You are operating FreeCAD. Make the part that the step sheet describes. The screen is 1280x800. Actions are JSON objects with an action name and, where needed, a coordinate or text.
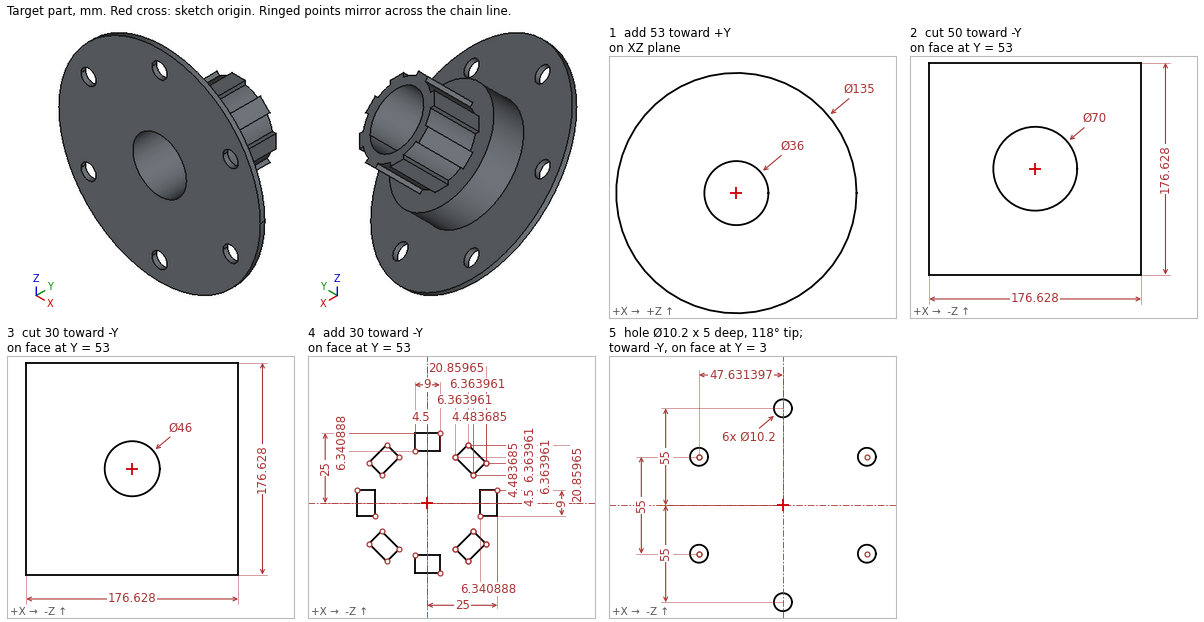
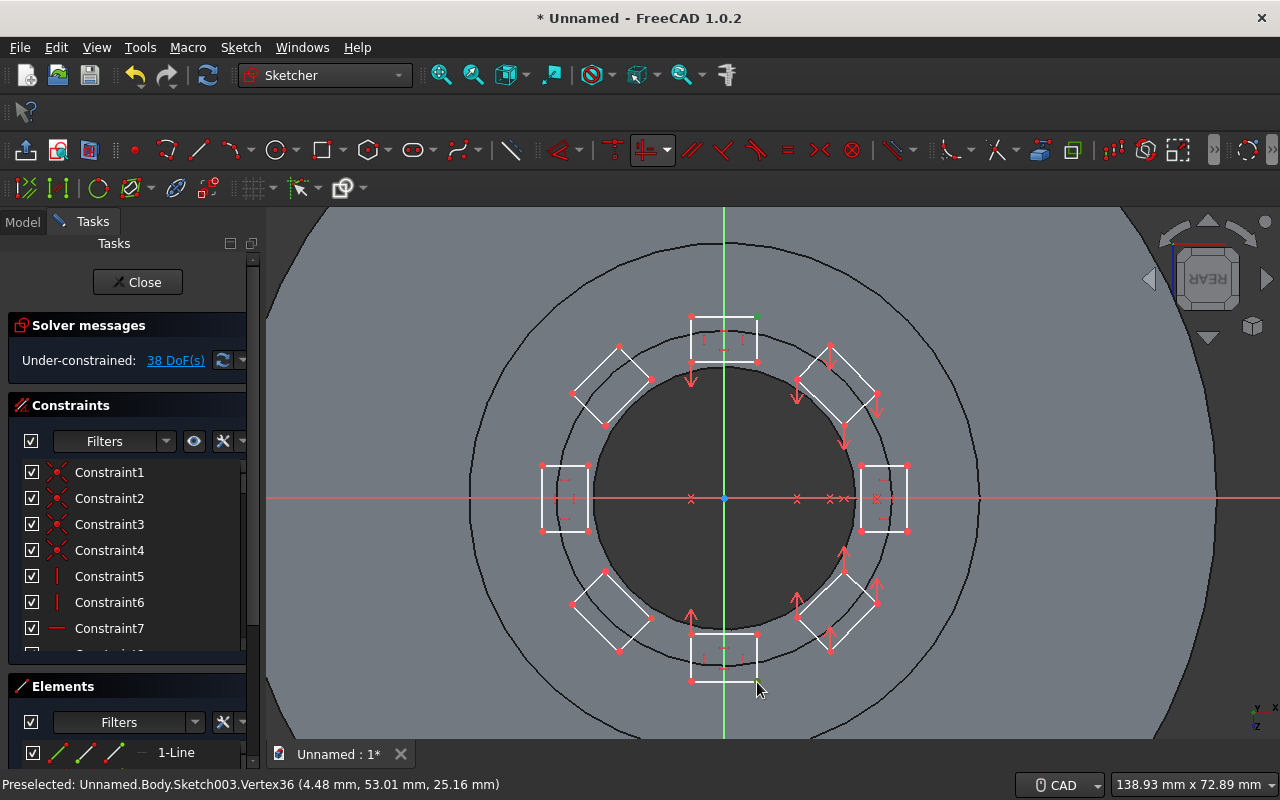
{"action": "left_click", "coordinate": [353, 498]}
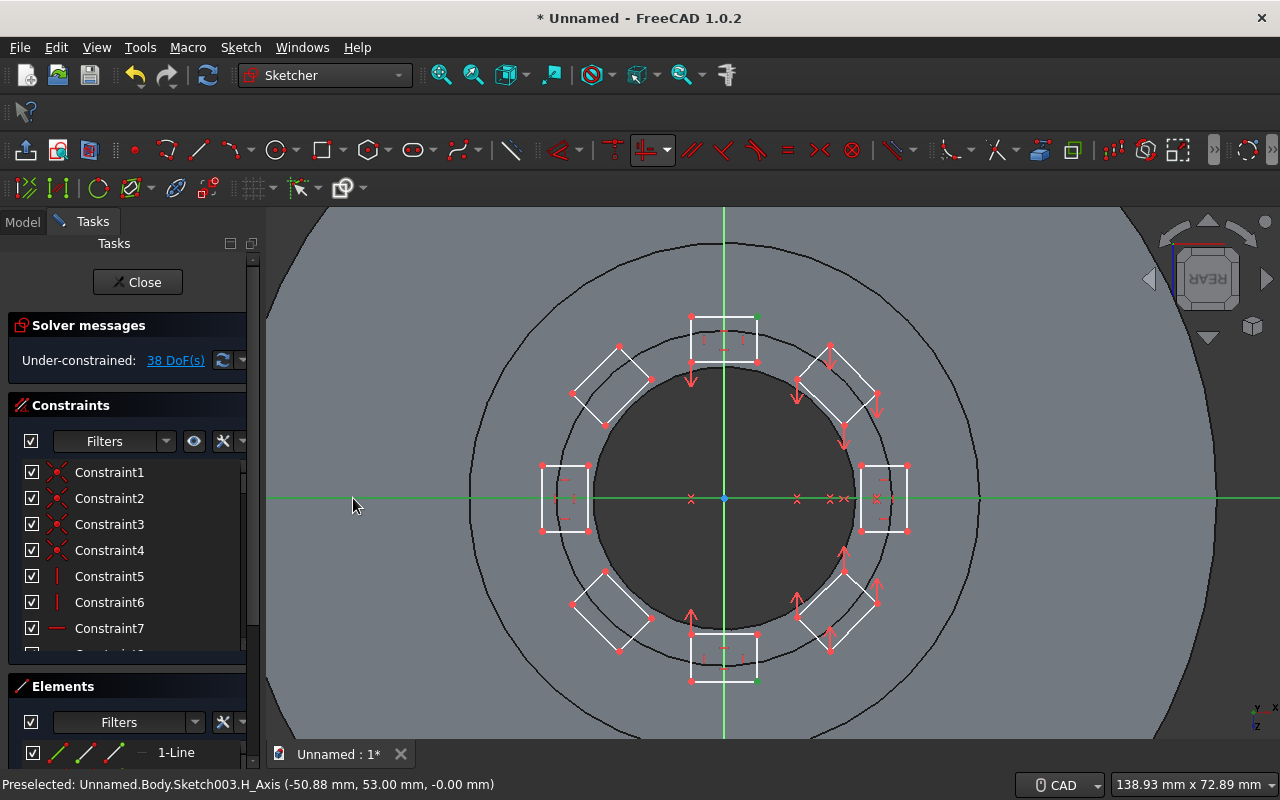
{"action": "left_click", "coordinate": [820, 150]}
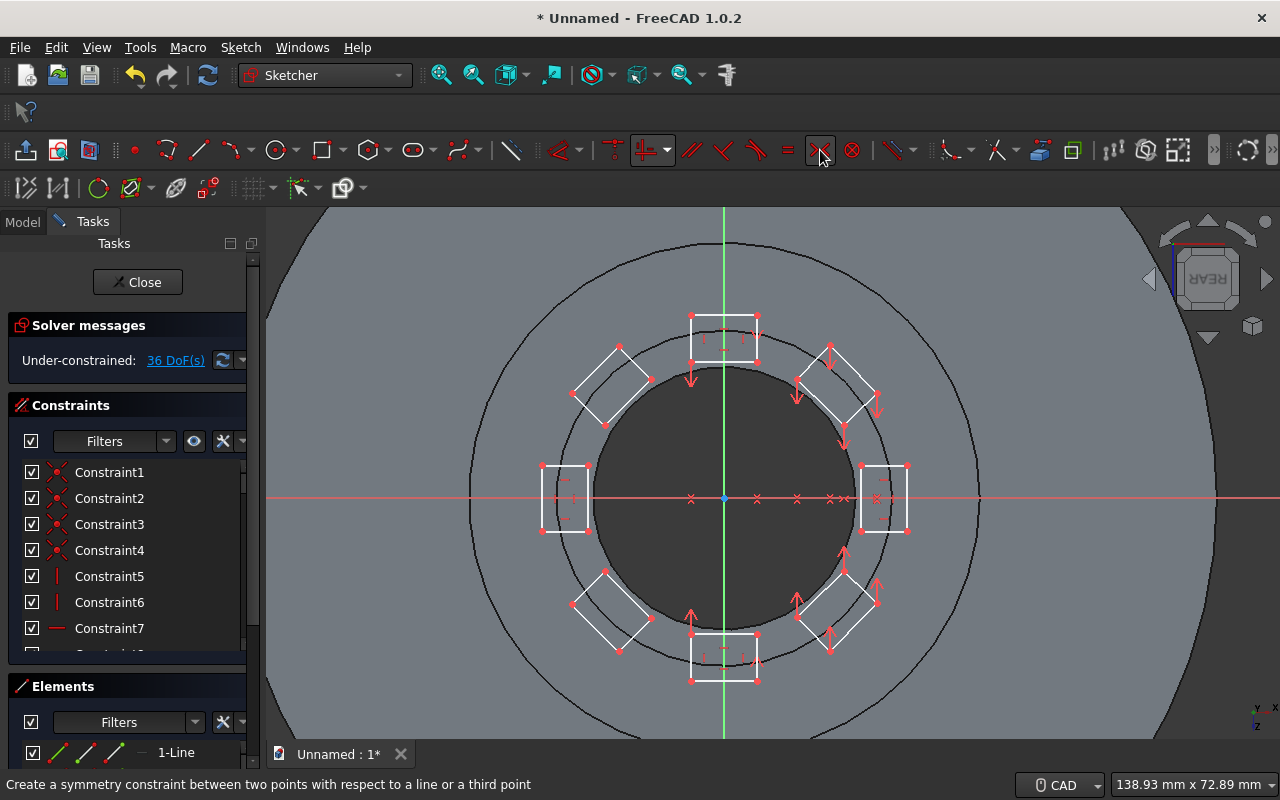
{"action": "left_click", "coordinate": [797, 617]}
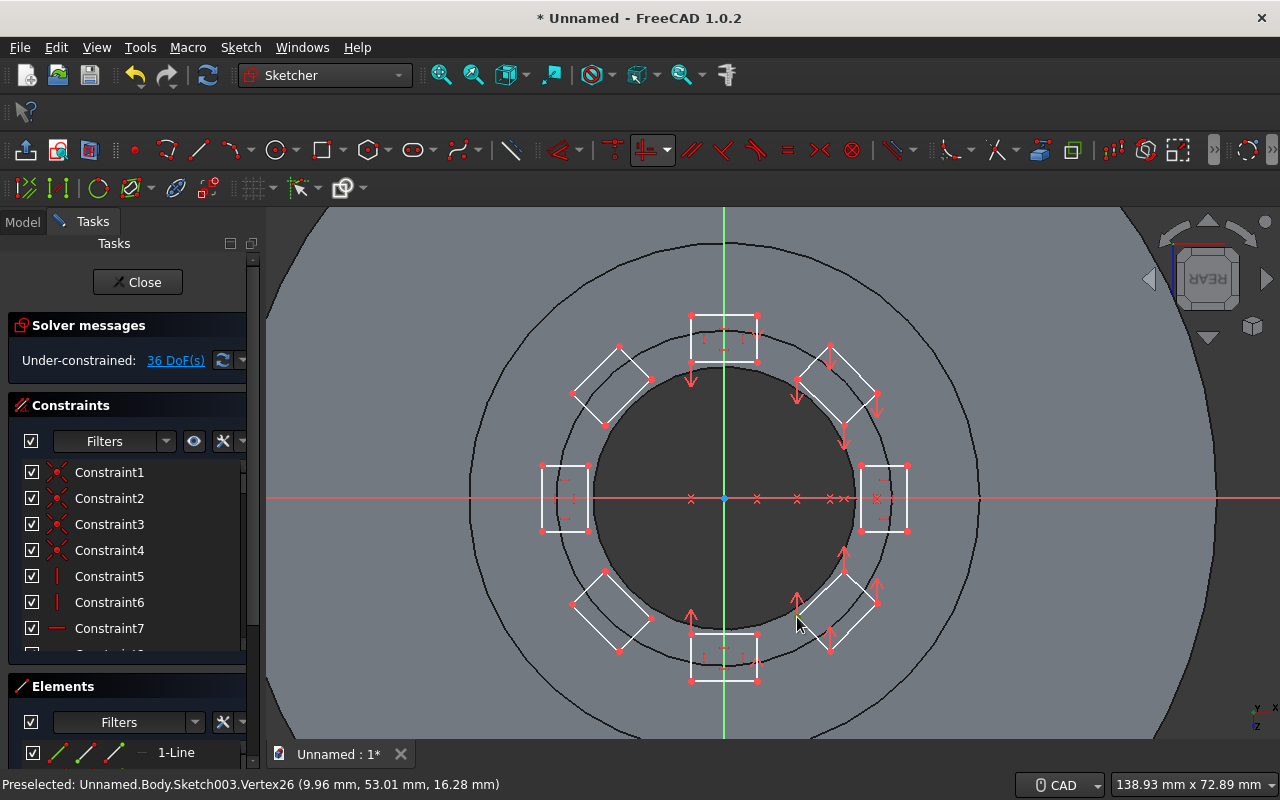
{"action": "left_click", "coordinate": [651, 619]}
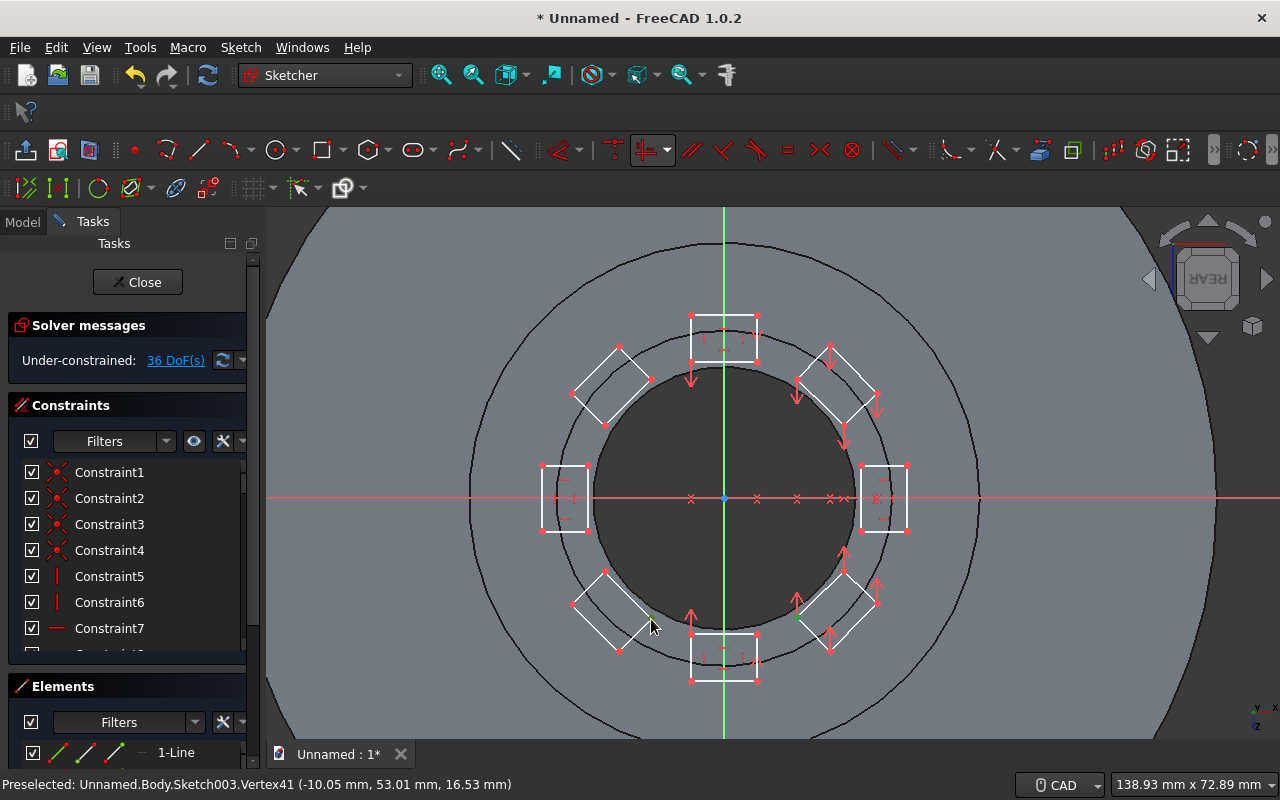
{"action": "left_click", "coordinate": [724, 575]}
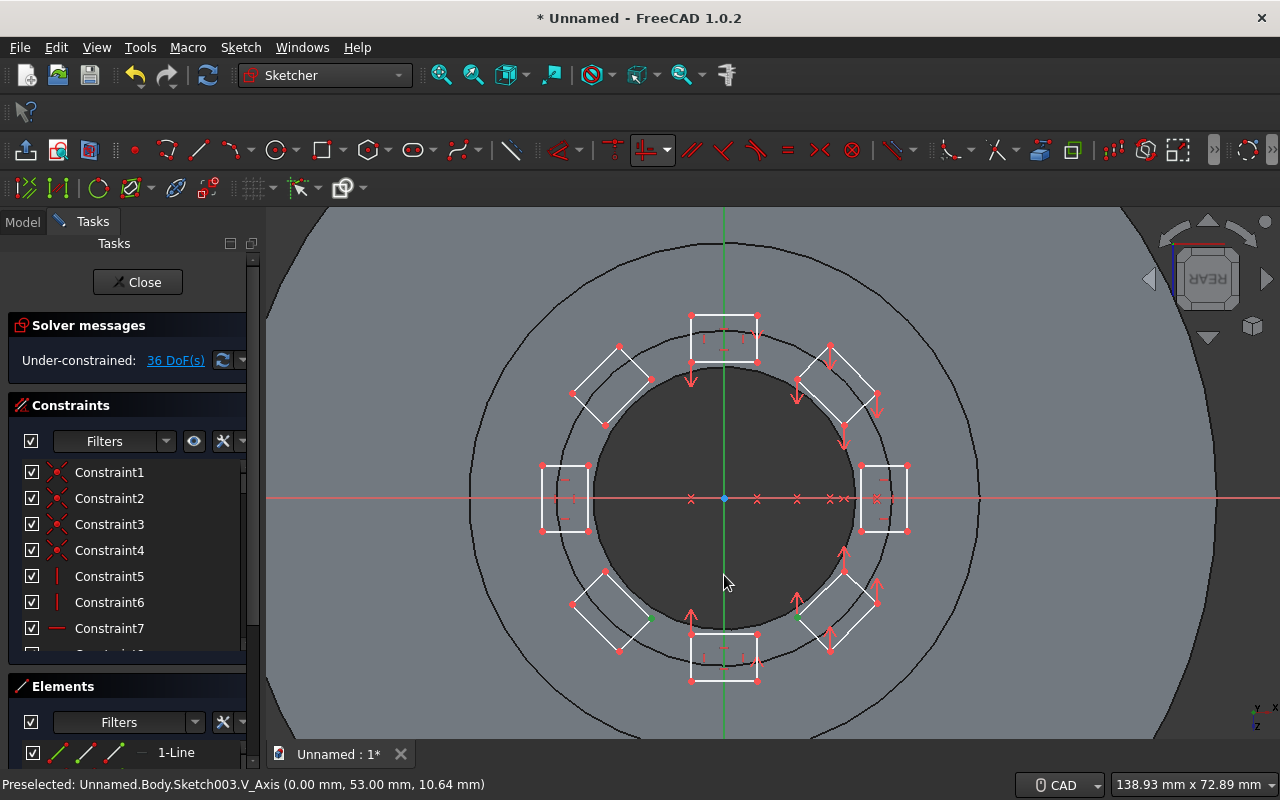
{"action": "left_click", "coordinate": [820, 150]}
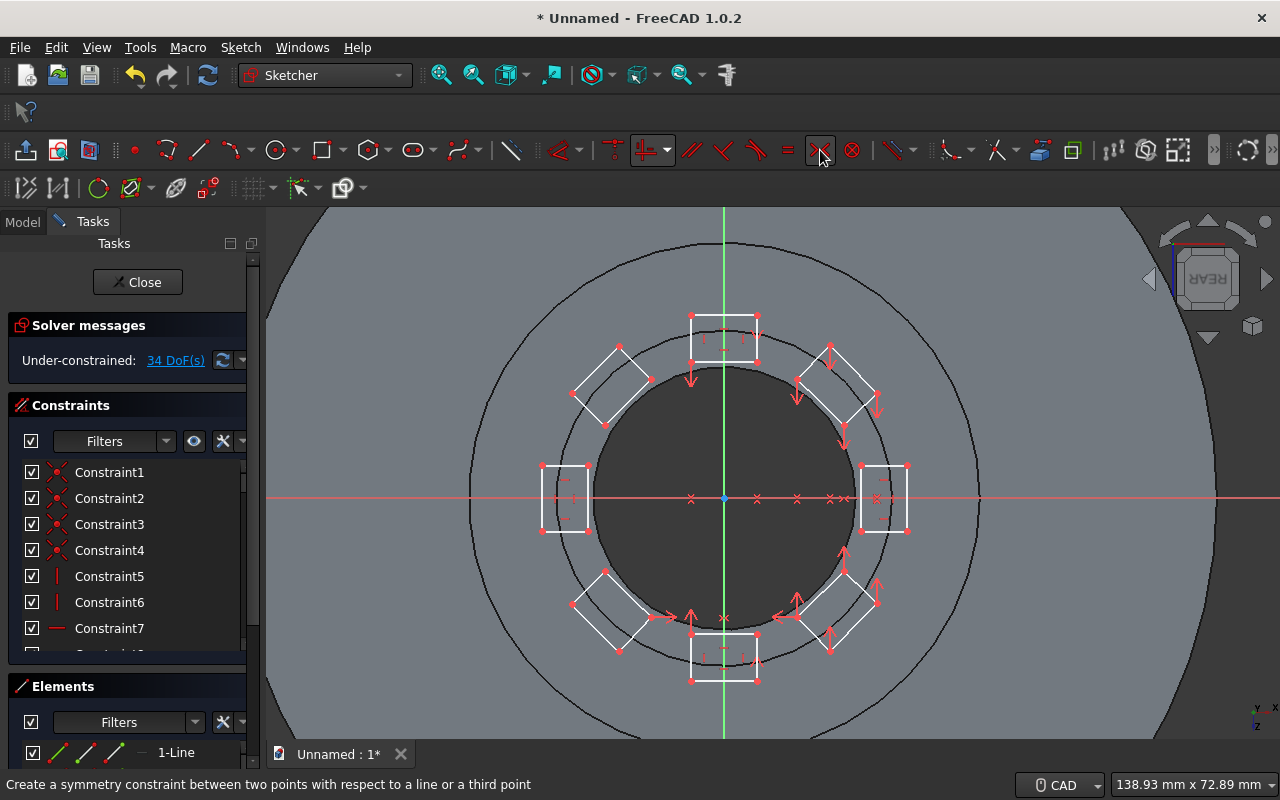
{"action": "left_click", "coordinate": [844, 571]}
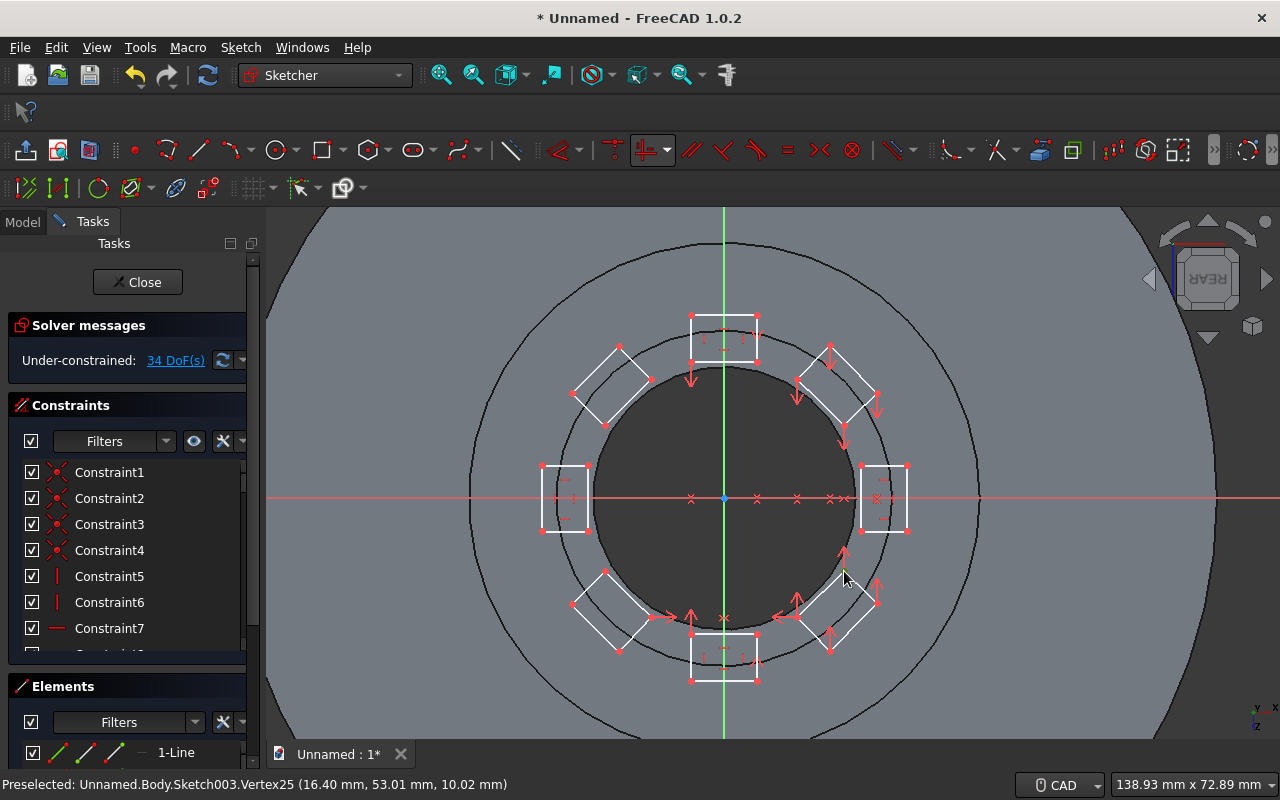
{"action": "left_click", "coordinate": [605, 572]}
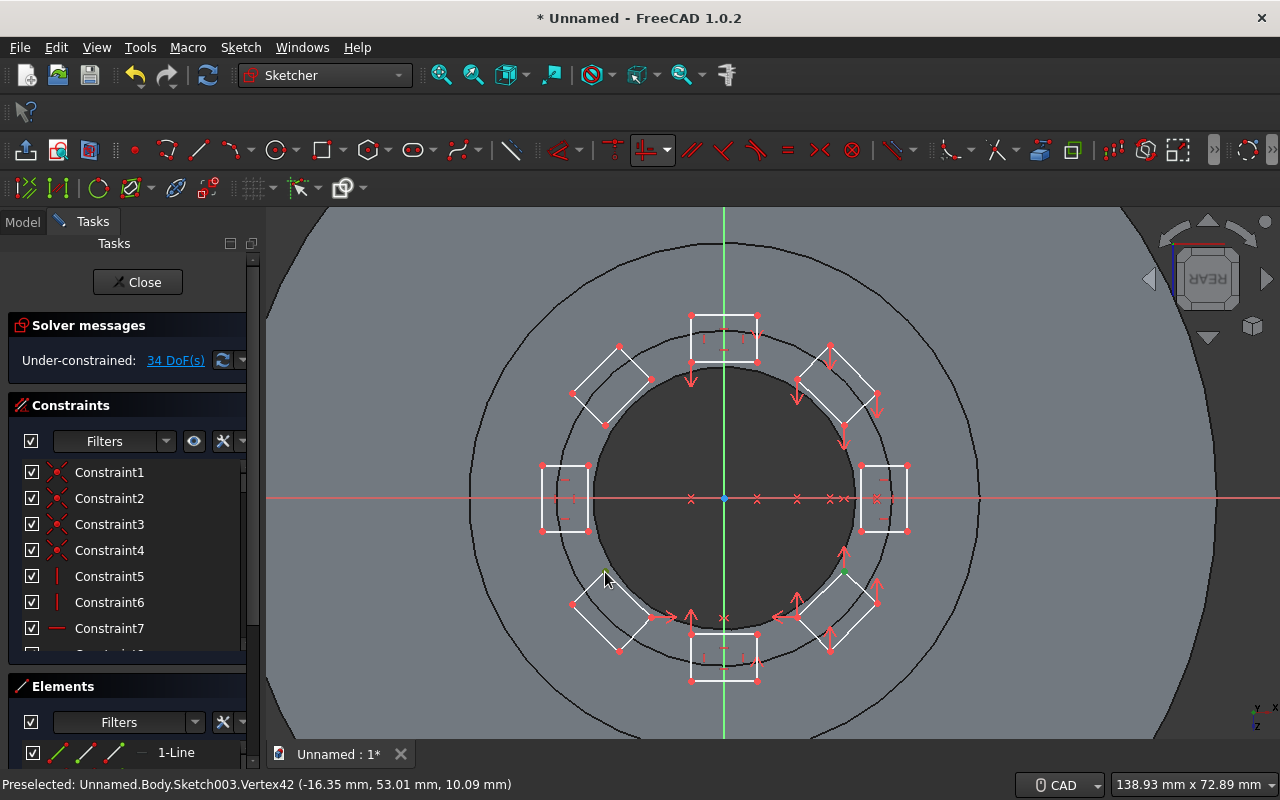
{"action": "left_click", "coordinate": [724, 575]}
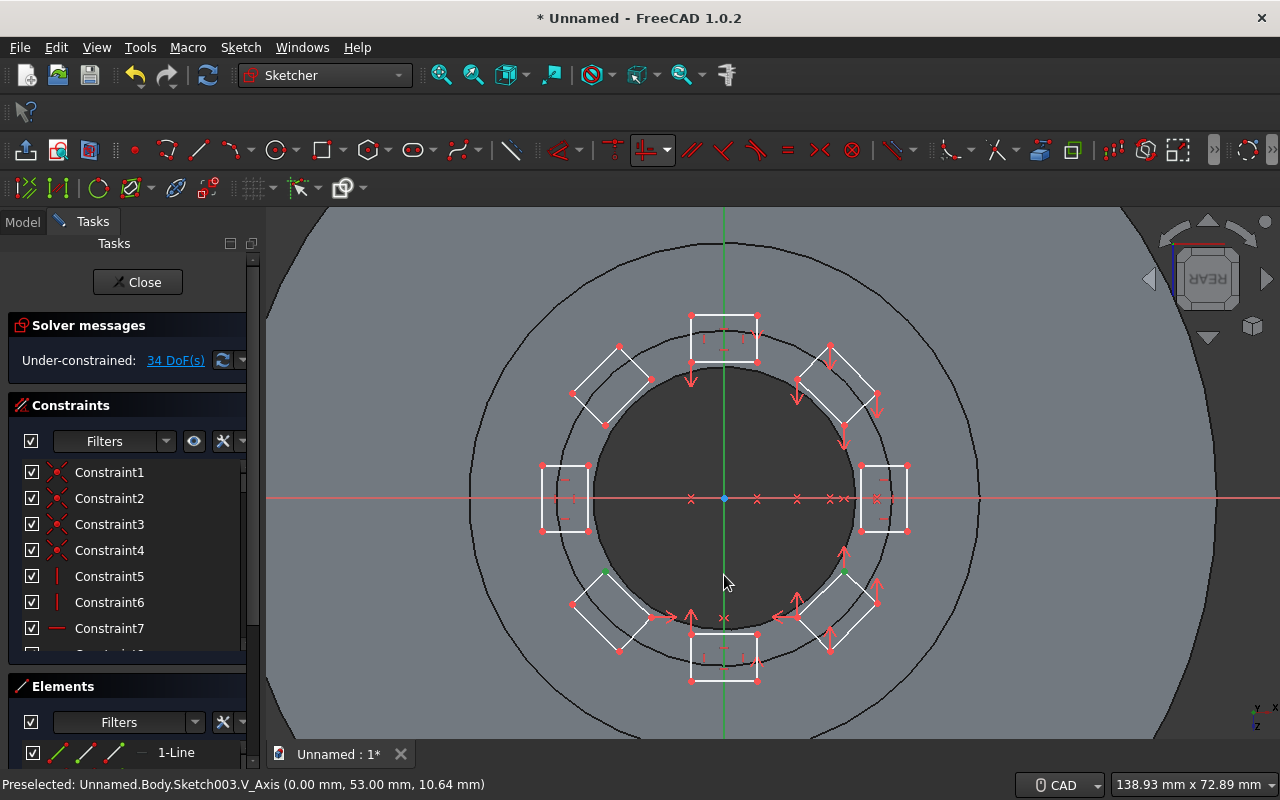
{"action": "left_click", "coordinate": [820, 150]}